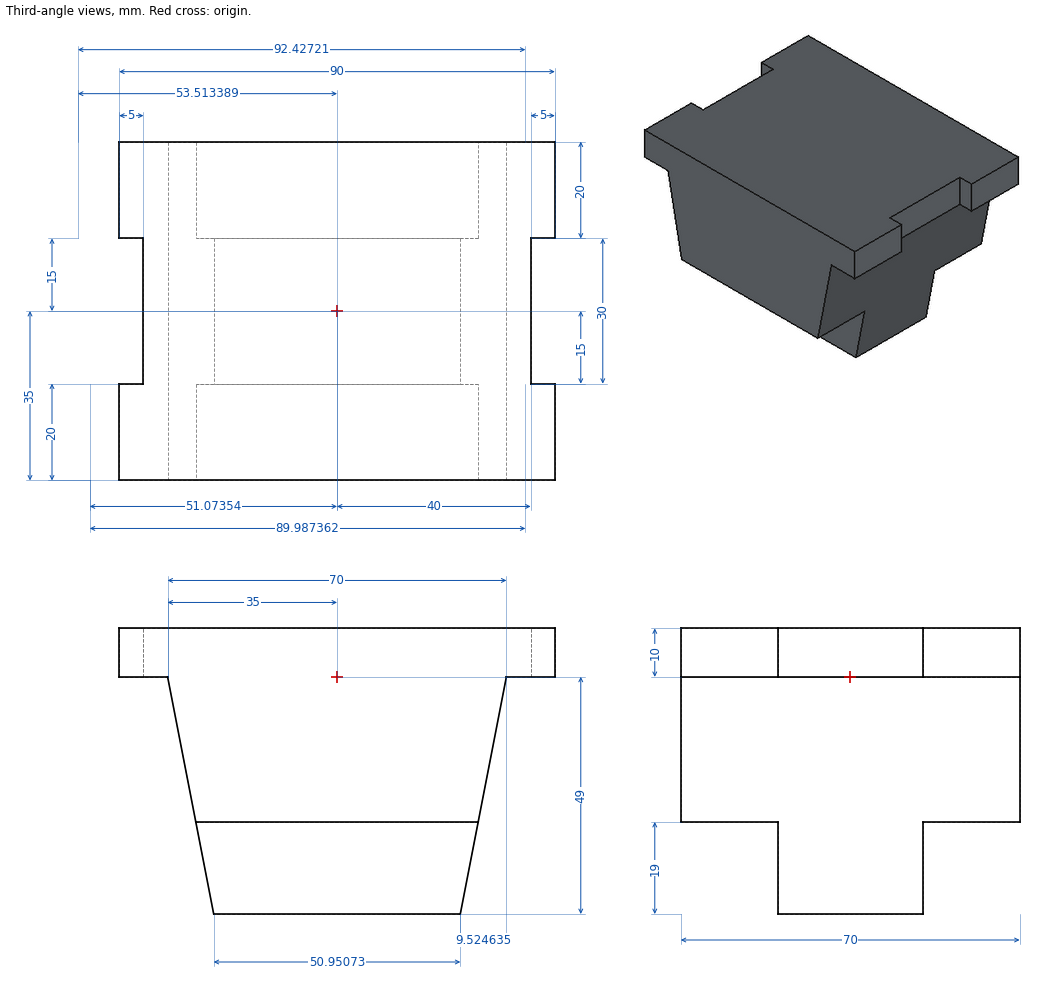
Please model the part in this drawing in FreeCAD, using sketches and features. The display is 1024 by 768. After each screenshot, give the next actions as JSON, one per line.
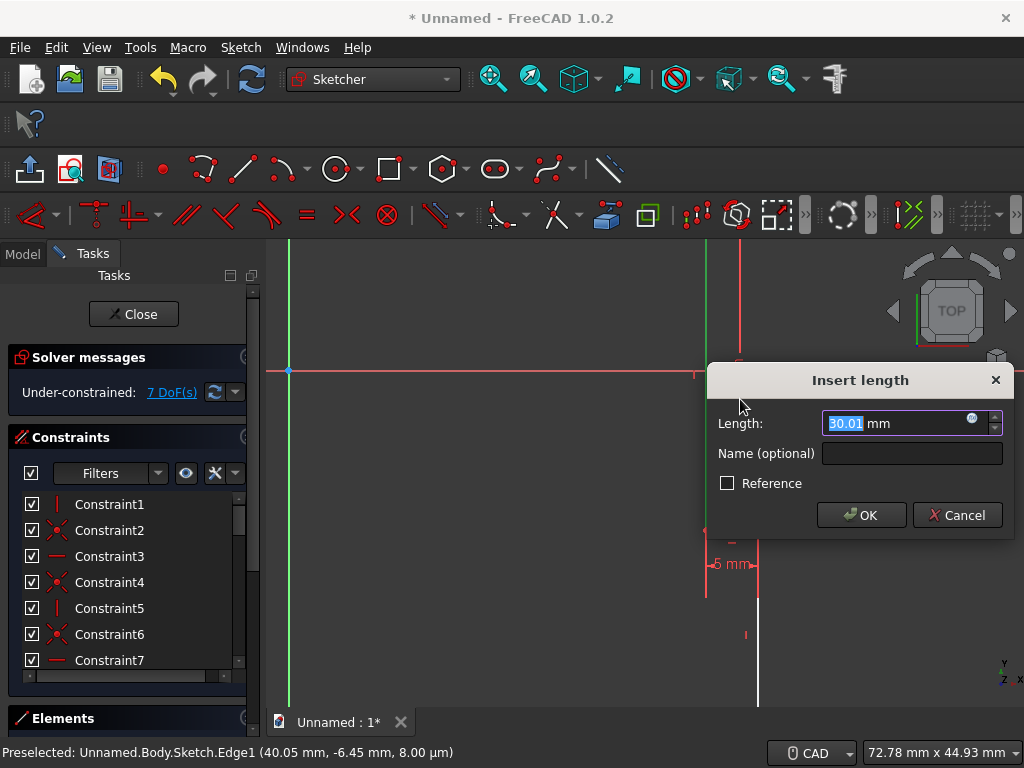
{"action": "type", "text": "30"}
{"action": "key", "text": "Return"}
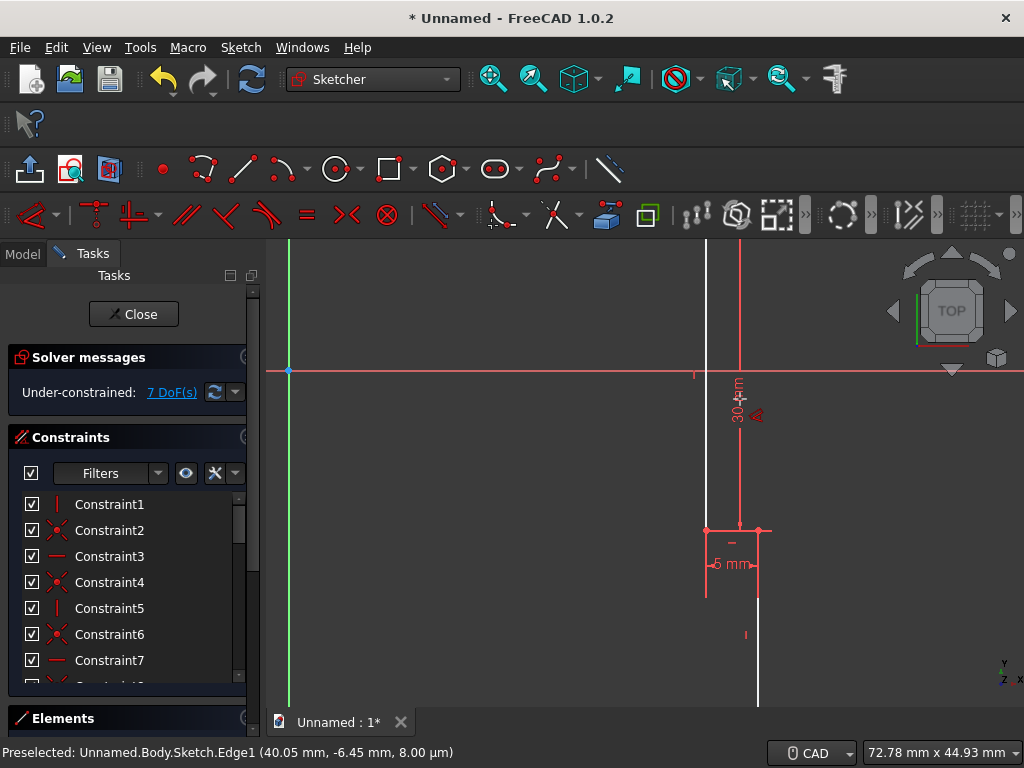
{"action": "scroll", "coordinate": [744, 532], "scroll_direction": "down", "scroll_amount": 5}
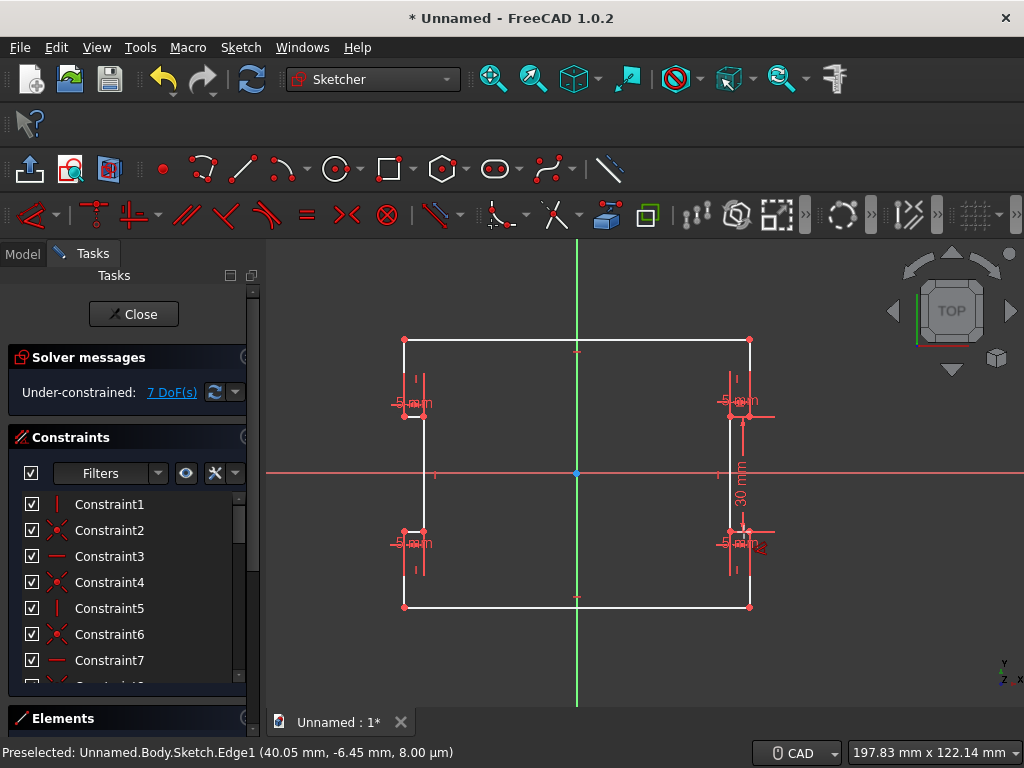
{"action": "left_click", "coordinate": [750, 394]}
{"action": "left_click", "coordinate": [784, 379]}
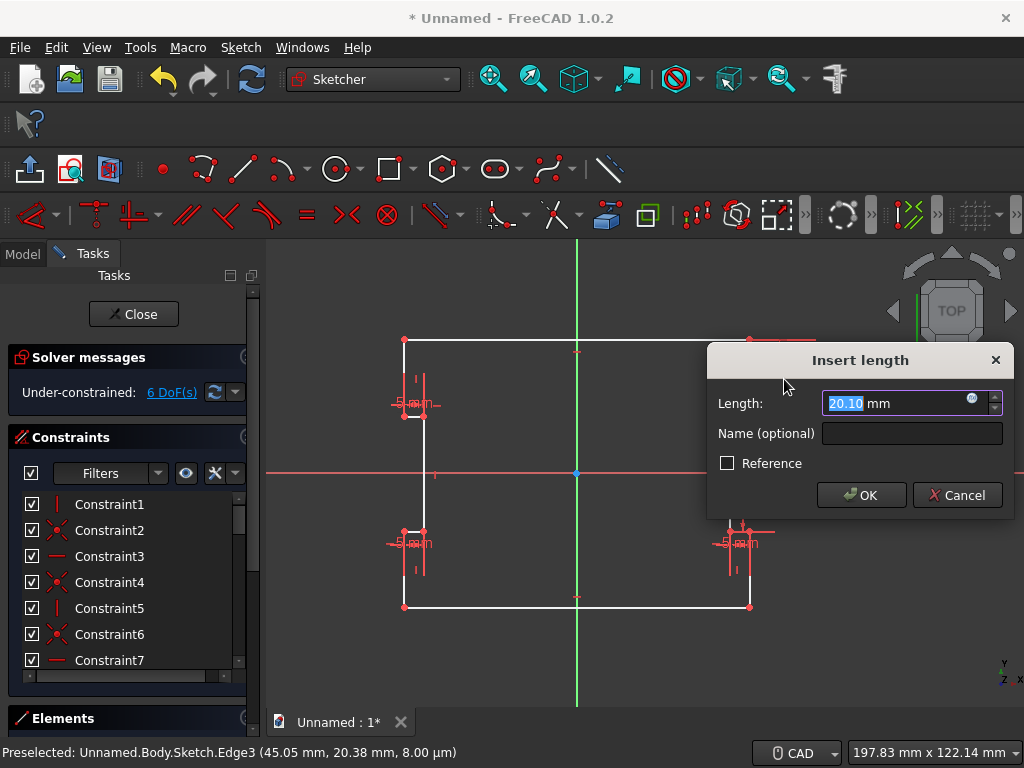
{"action": "type", "text": "20"}
{"action": "key", "text": "Return"}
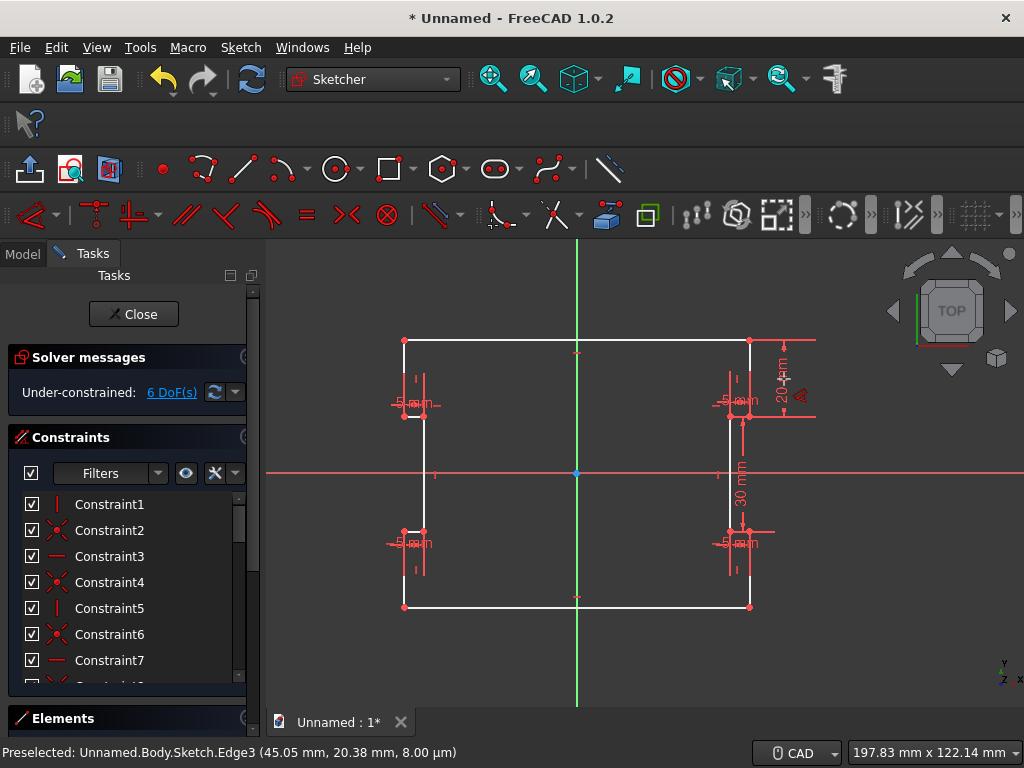
{"action": "left_click", "coordinate": [646, 340]}
{"action": "left_click", "coordinate": [498, 306]}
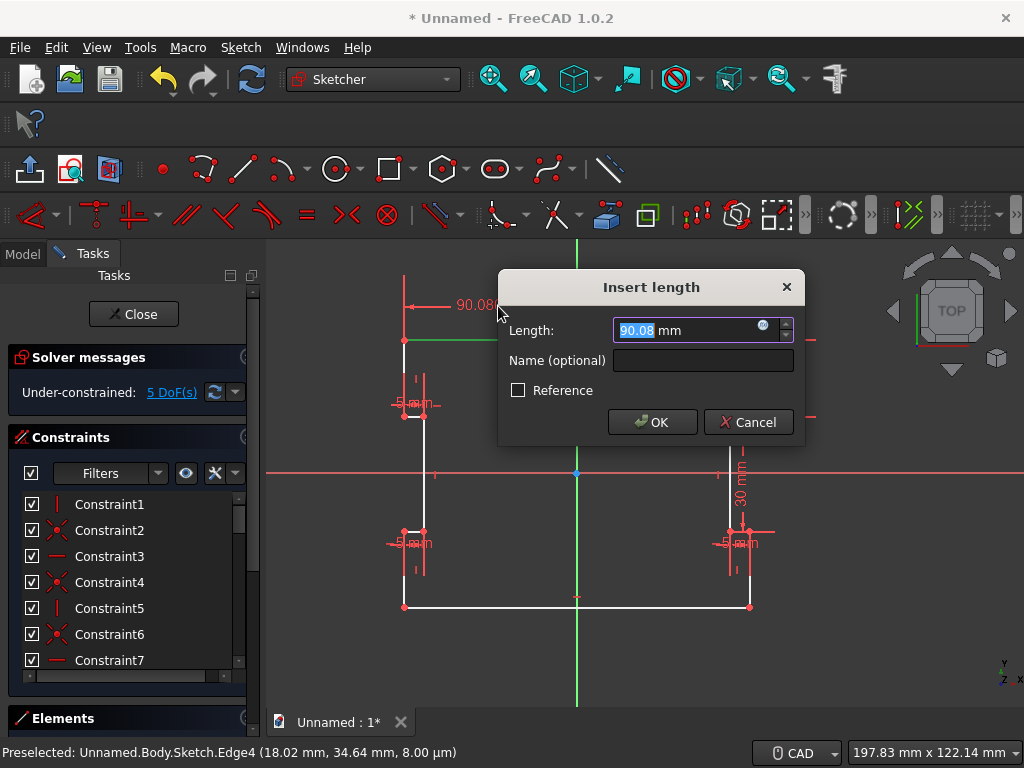
{"action": "type", "text": "90"}
{"action": "key", "text": "Return"}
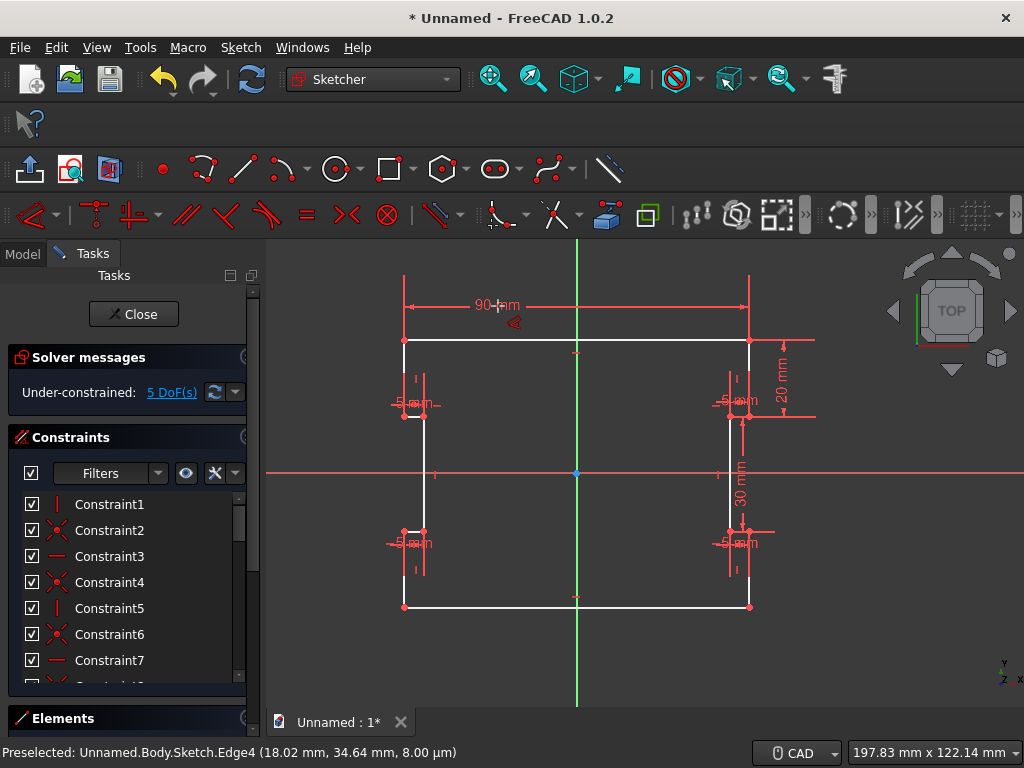
{"action": "left_click", "coordinate": [404, 363]}
{"action": "left_click", "coordinate": [370, 379]}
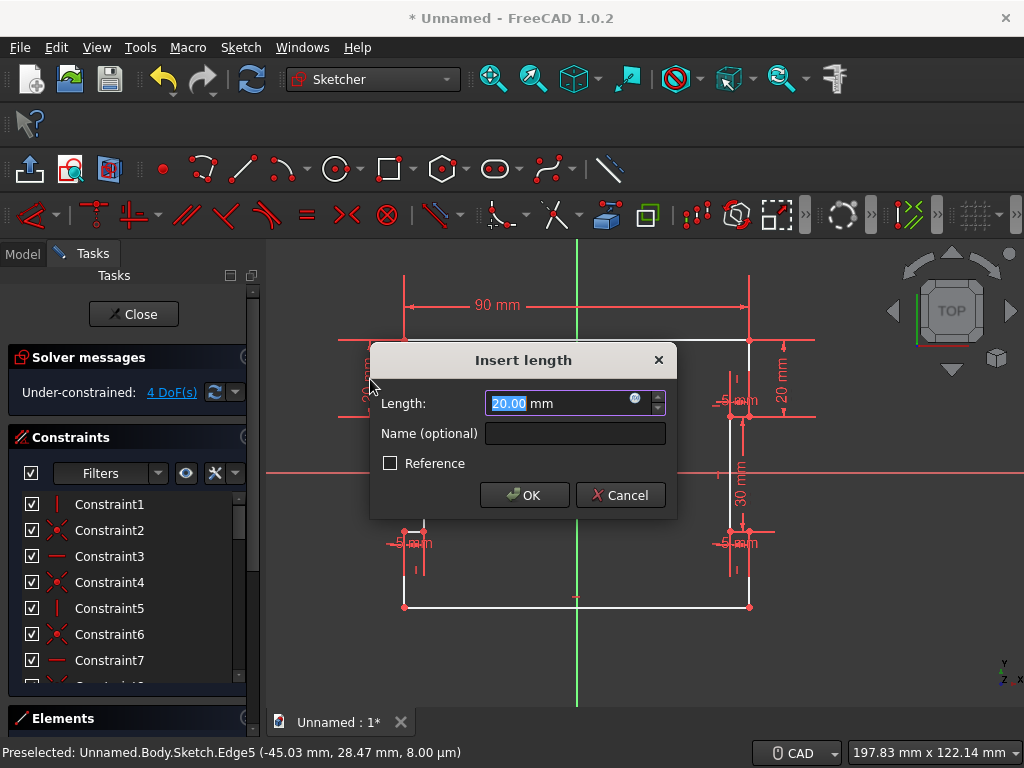
{"action": "type", "text": "20"}
{"action": "key", "text": "Return"}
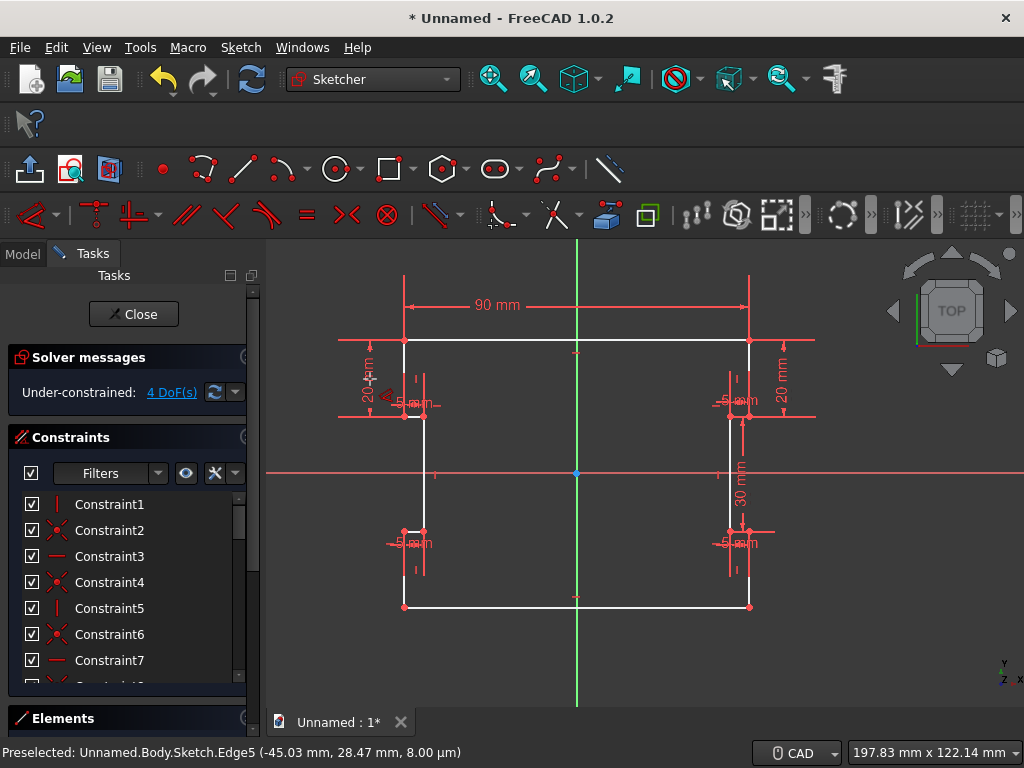
{"action": "left_click", "coordinate": [424, 452]}
{"action": "left_click", "coordinate": [390, 448]}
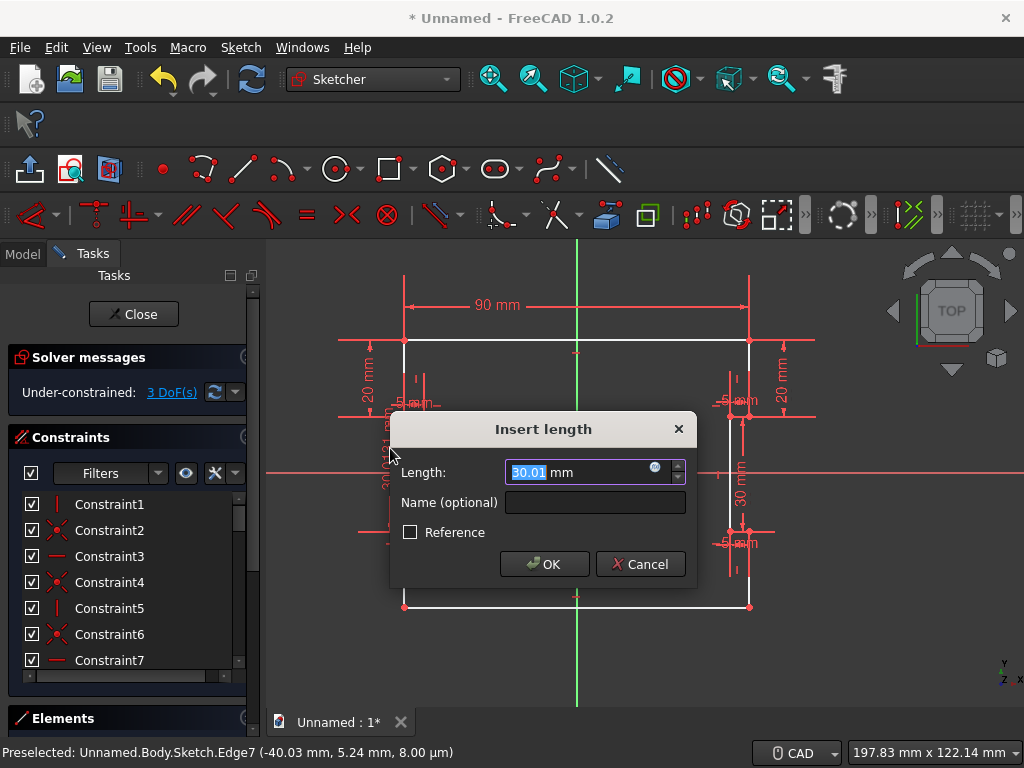
{"action": "type", "text": "30"}
{"action": "key", "text": "Return"}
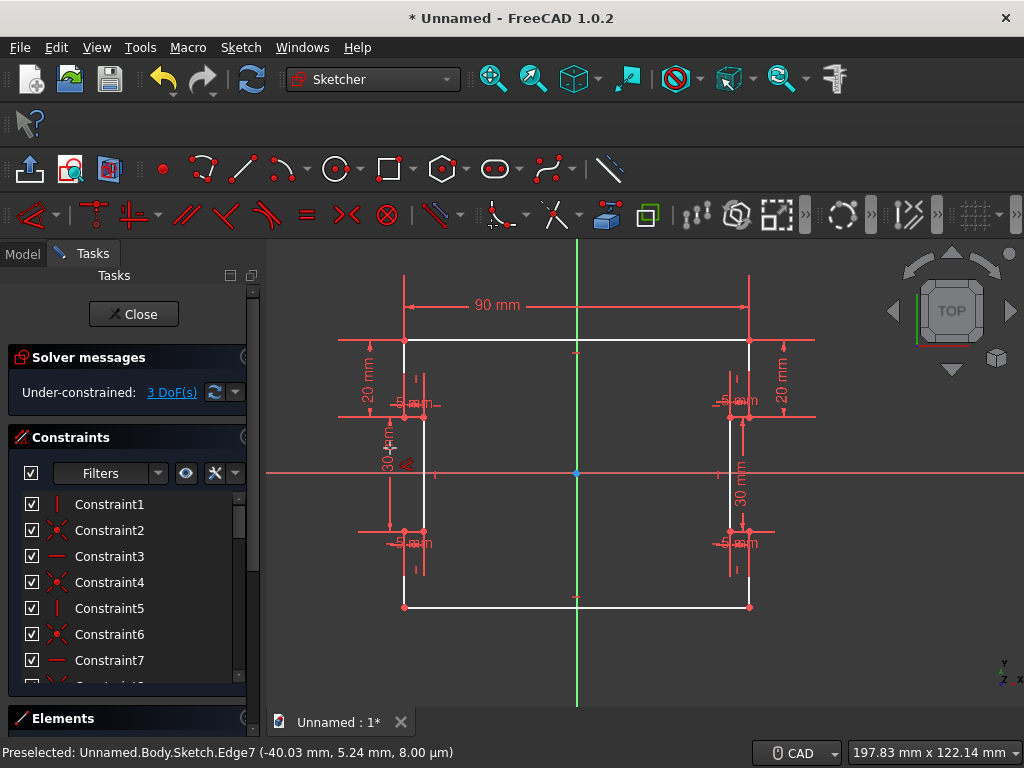
{"action": "left_click", "coordinate": [404, 555]}
{"action": "left_click", "coordinate": [370, 570]}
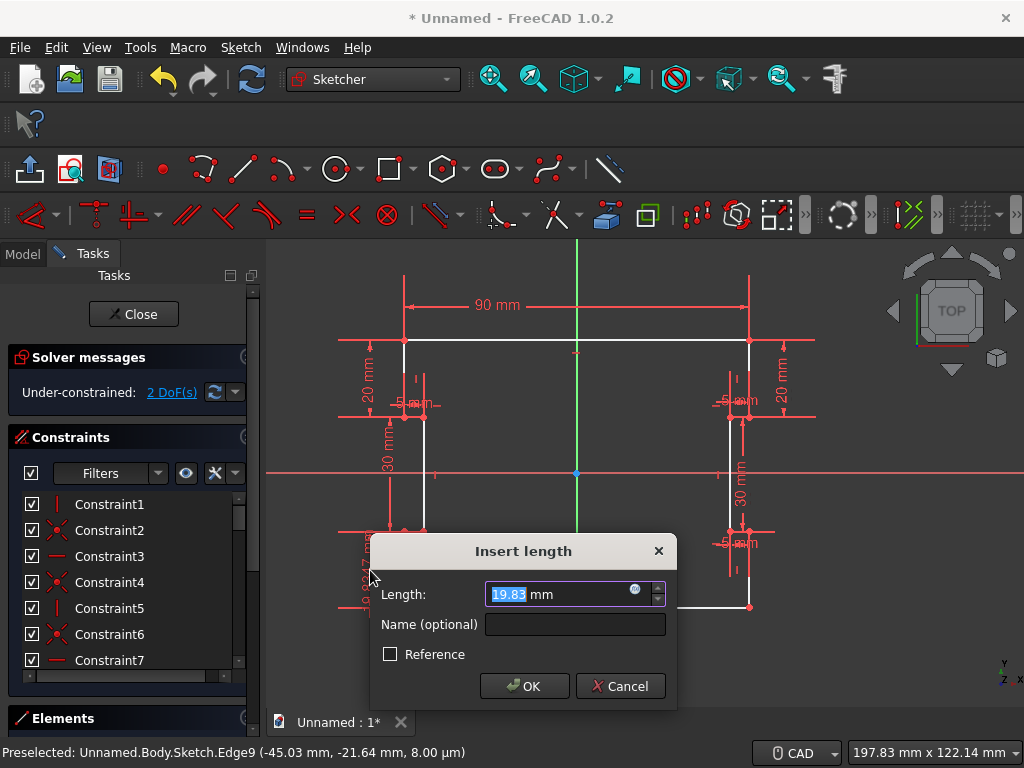
{"action": "type", "text": "20"}
{"action": "key", "text": "Return"}